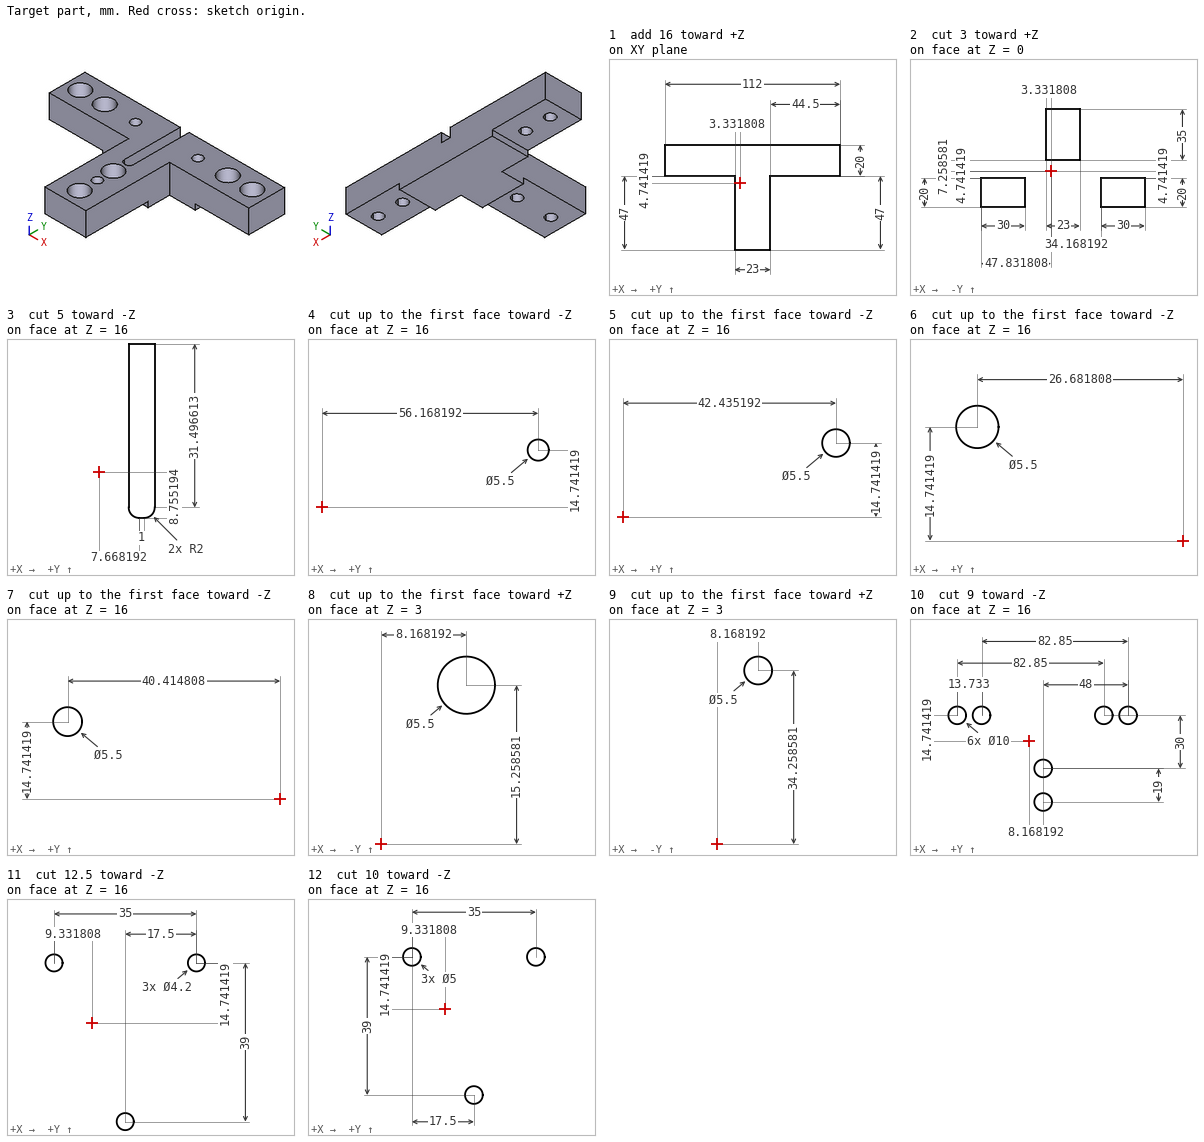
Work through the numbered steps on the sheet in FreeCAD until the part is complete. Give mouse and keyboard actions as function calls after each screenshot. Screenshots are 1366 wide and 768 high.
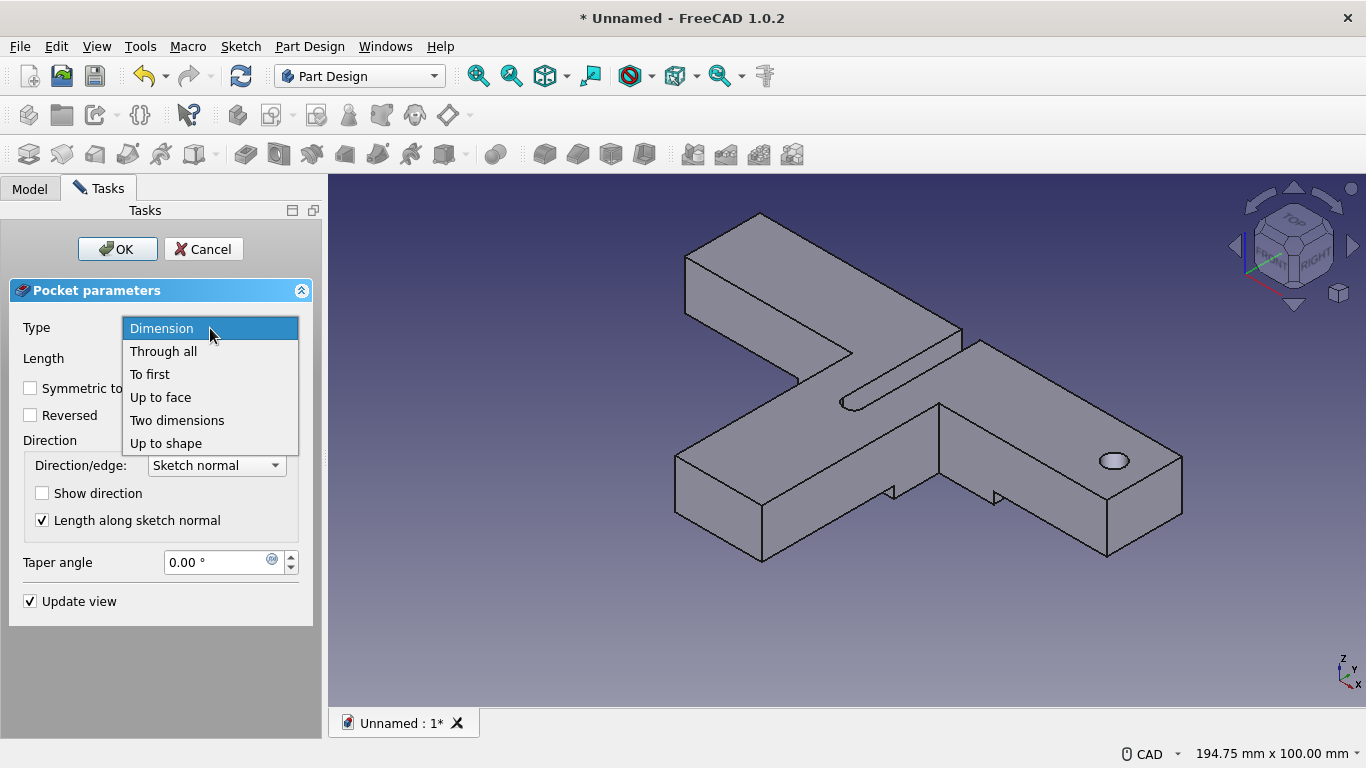
click(208, 374)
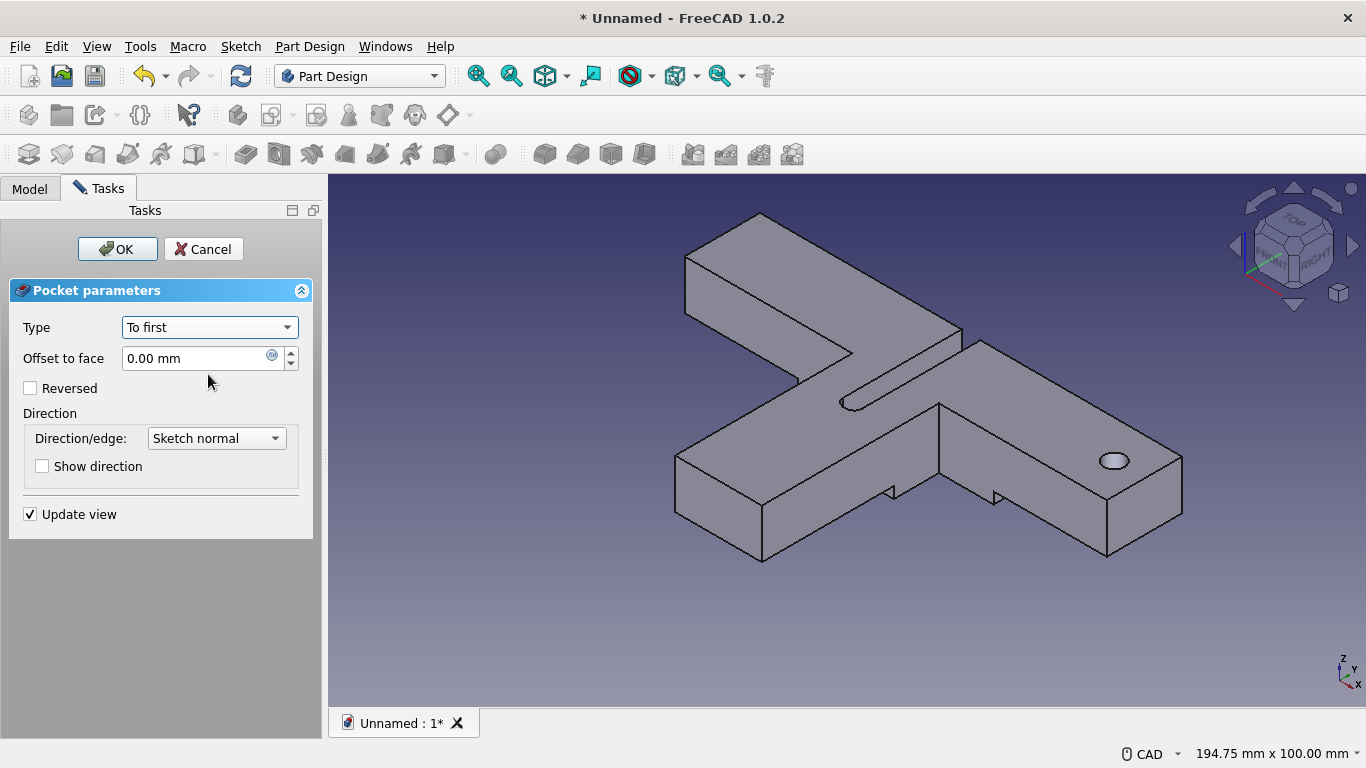
click(118, 249)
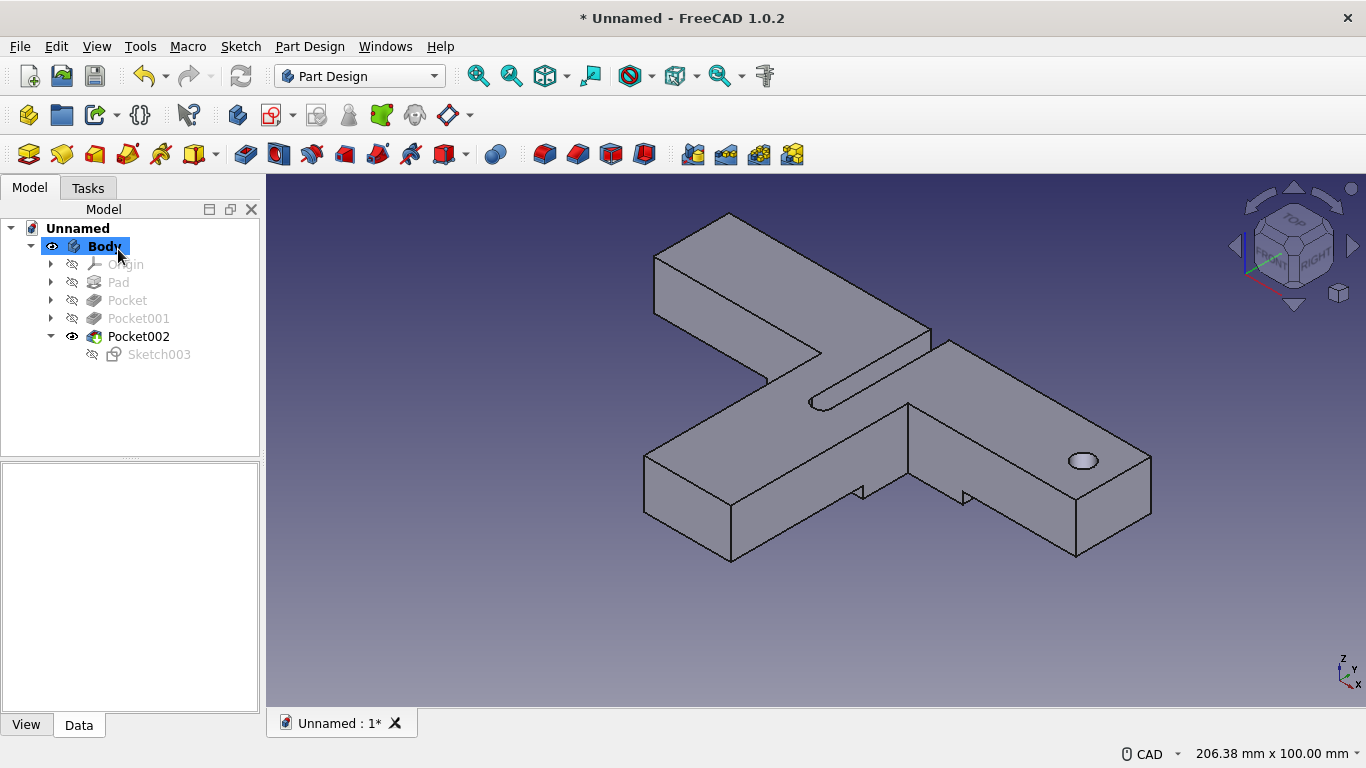
click(742, 448)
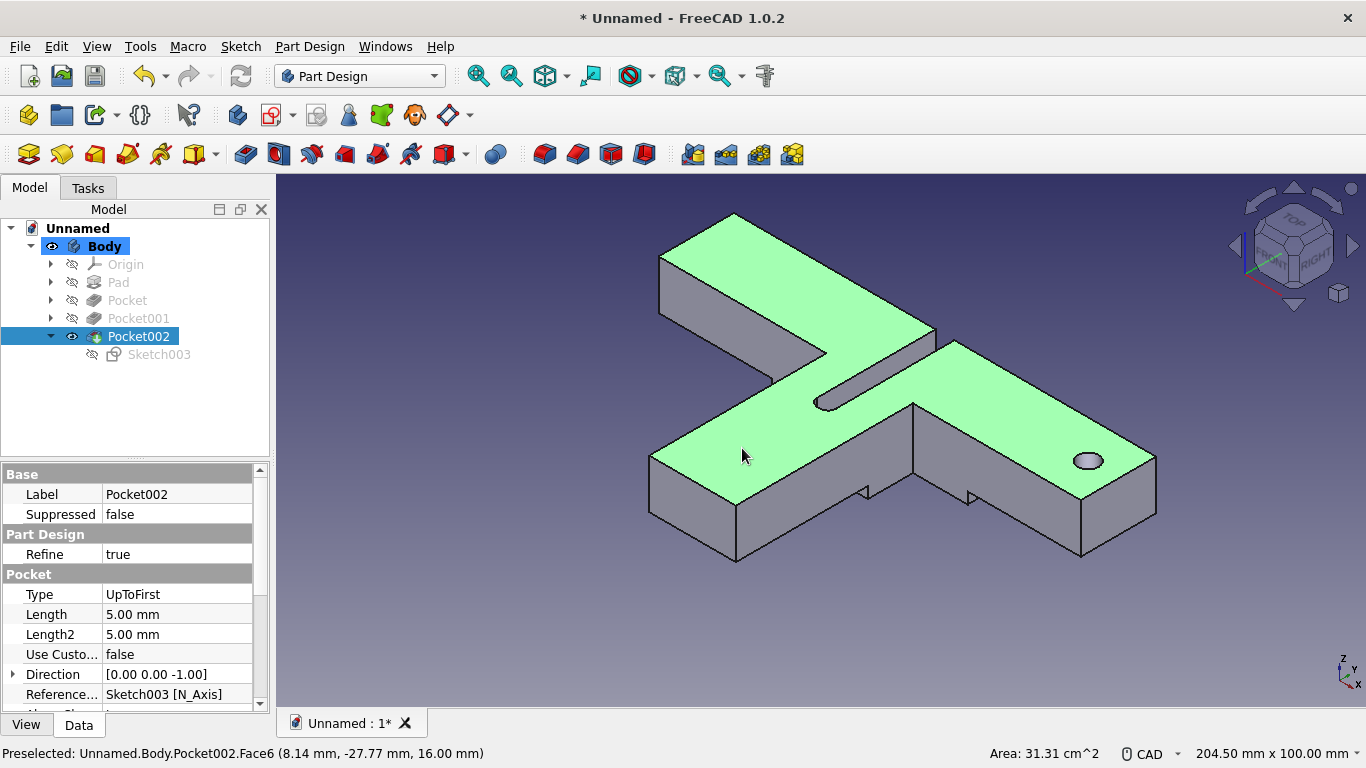
click(270, 116)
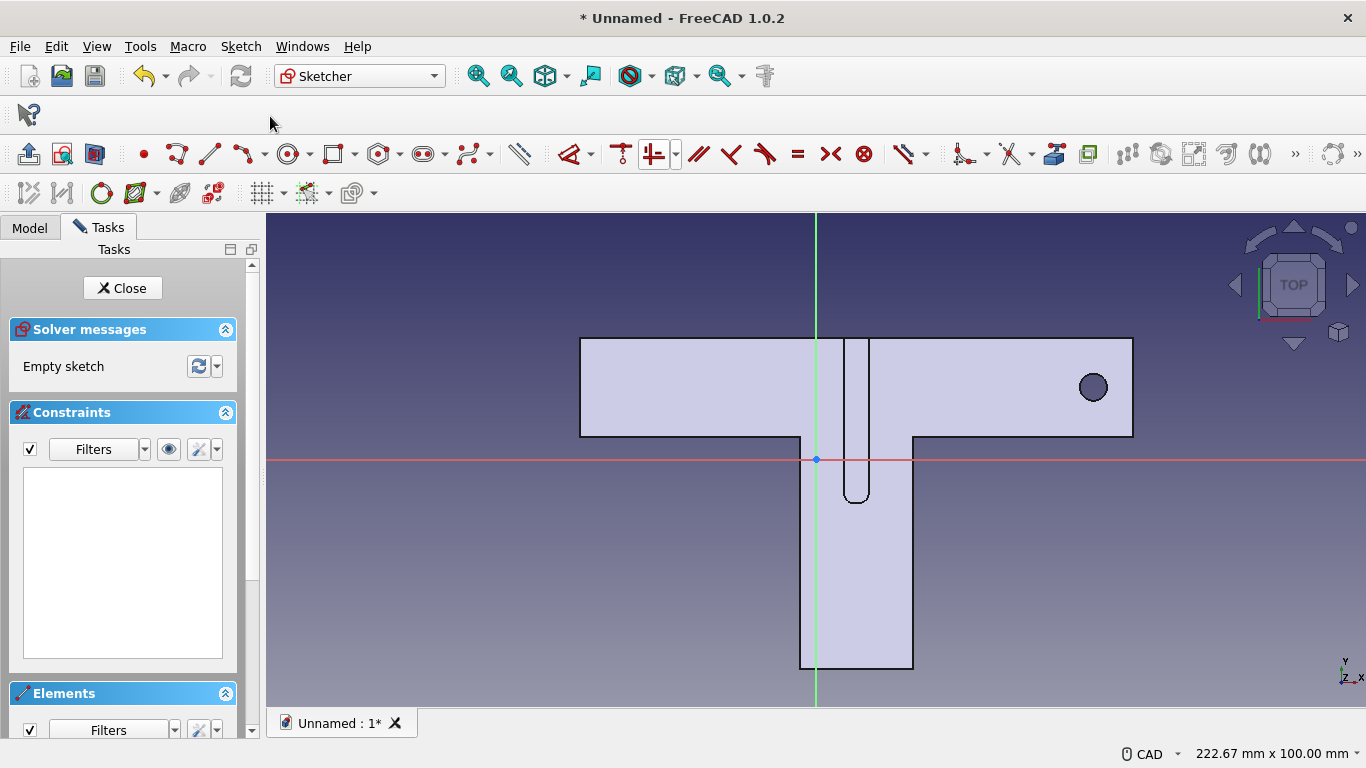
scroll(1053, 380, up, 12)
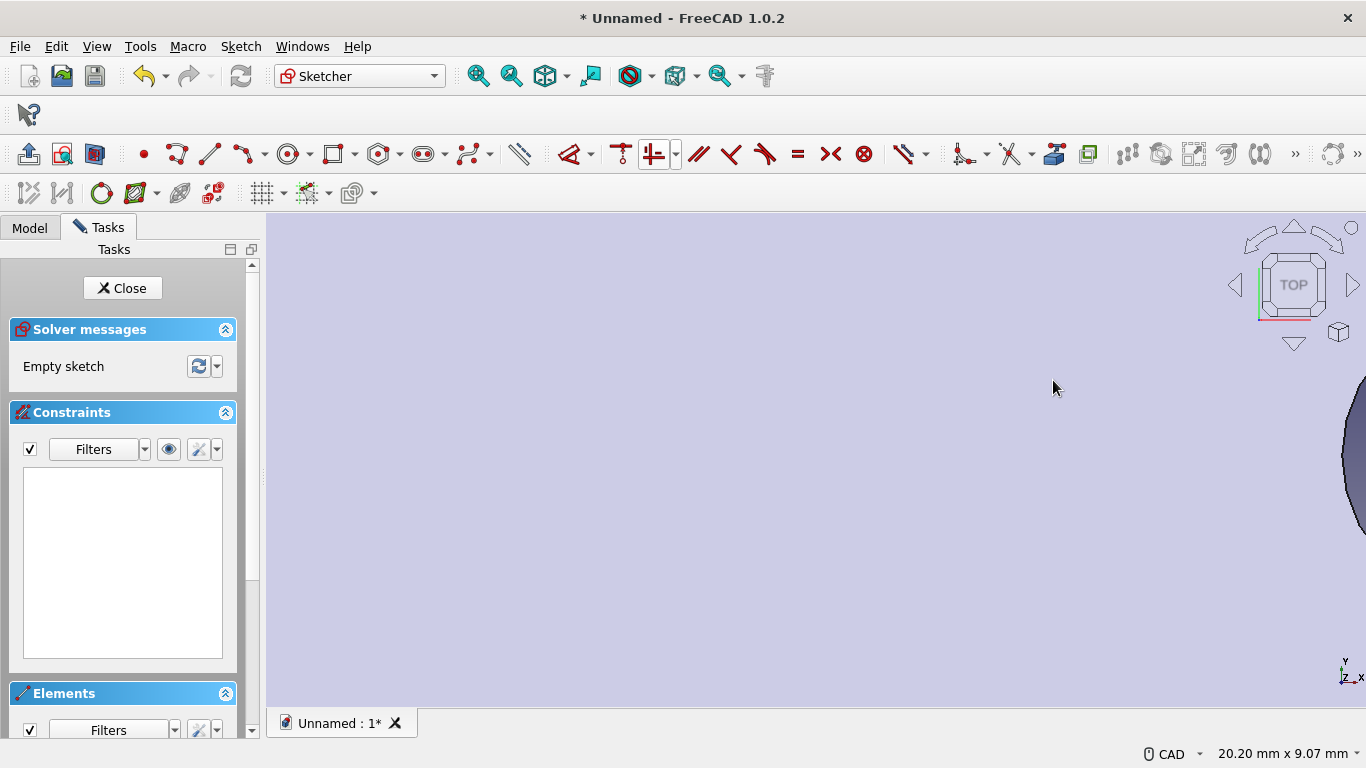
click(288, 154)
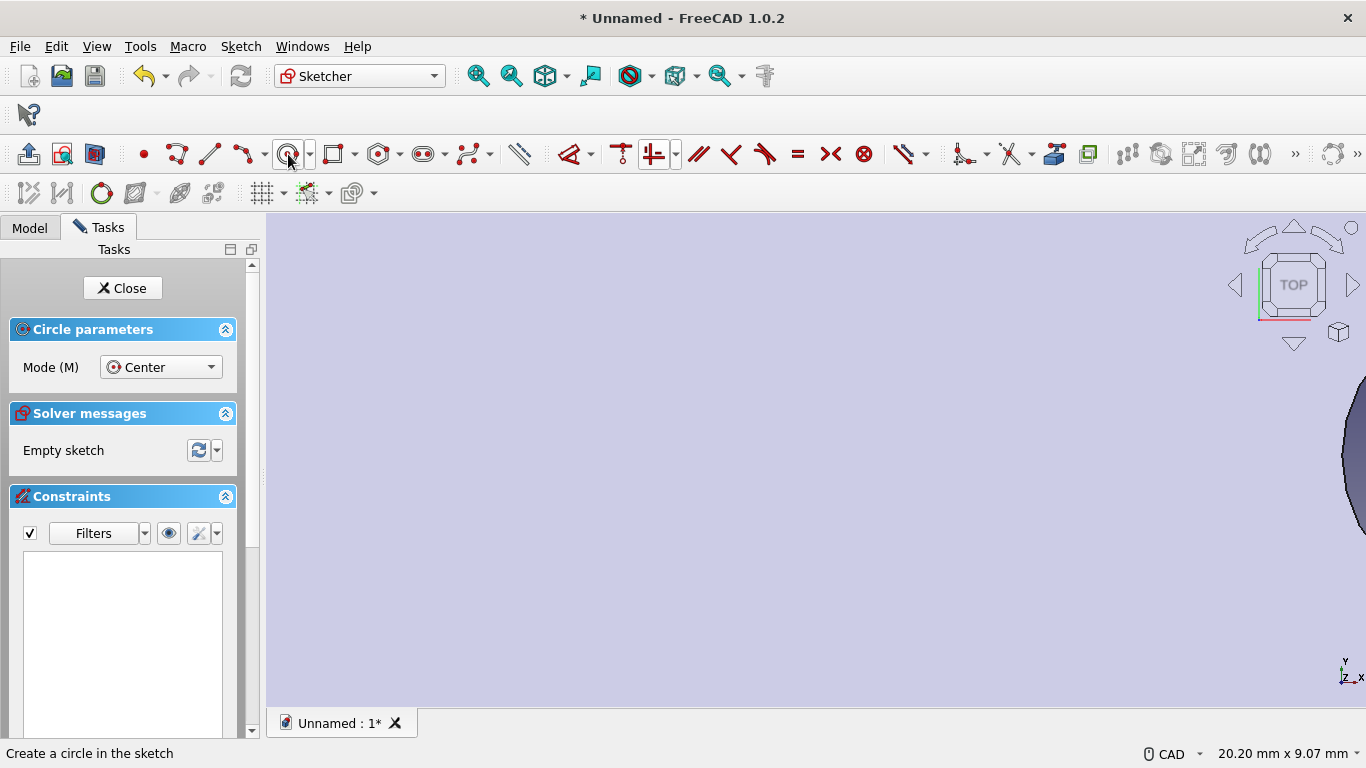
click(744, 456)
move(850, 350)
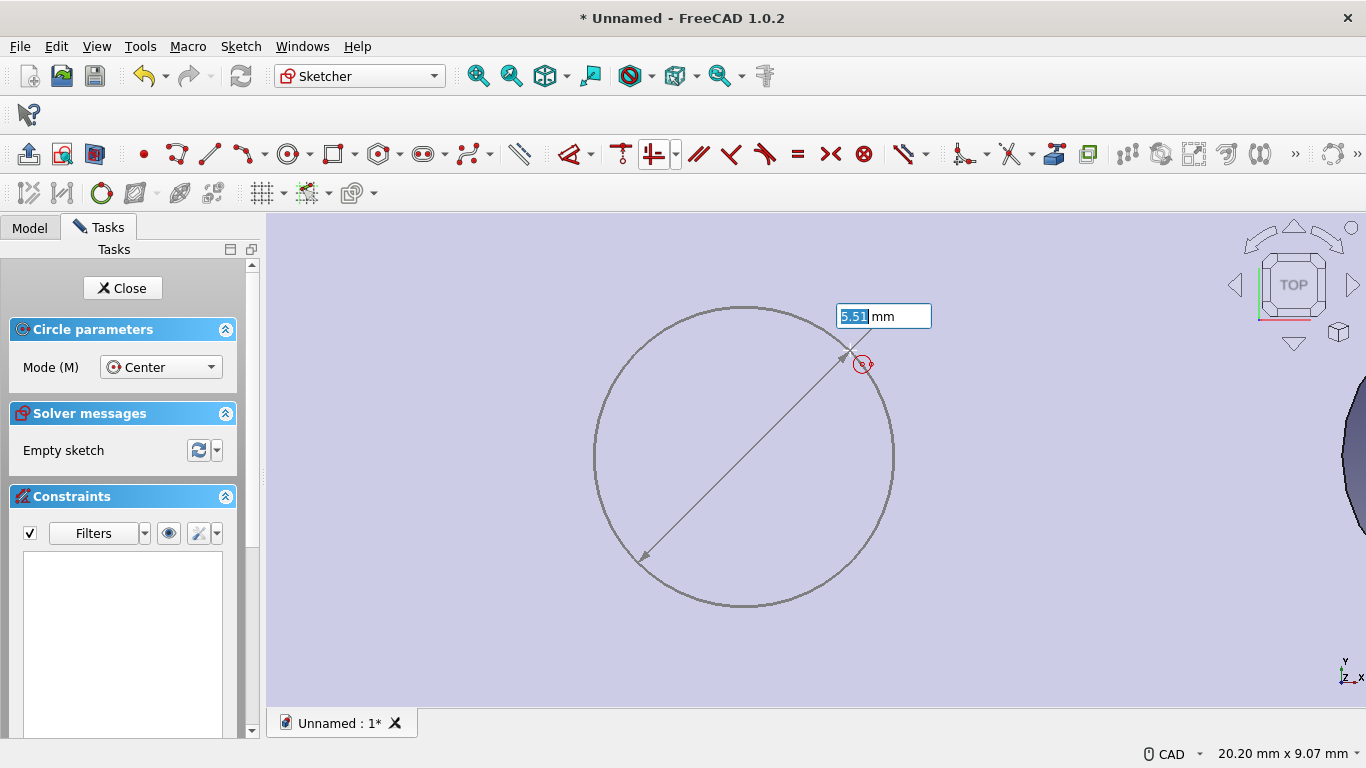
text(5.5)
key(Return)
key(Escape)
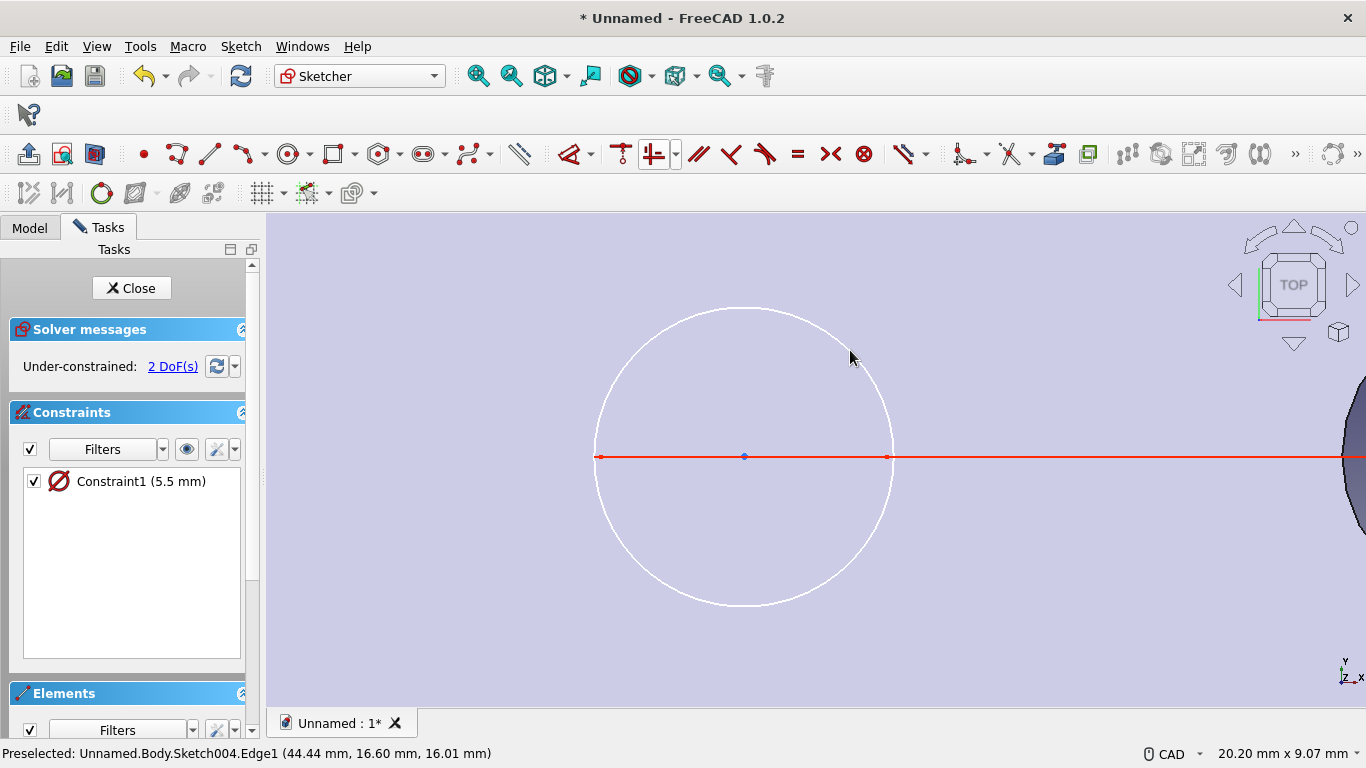
click(568, 154)